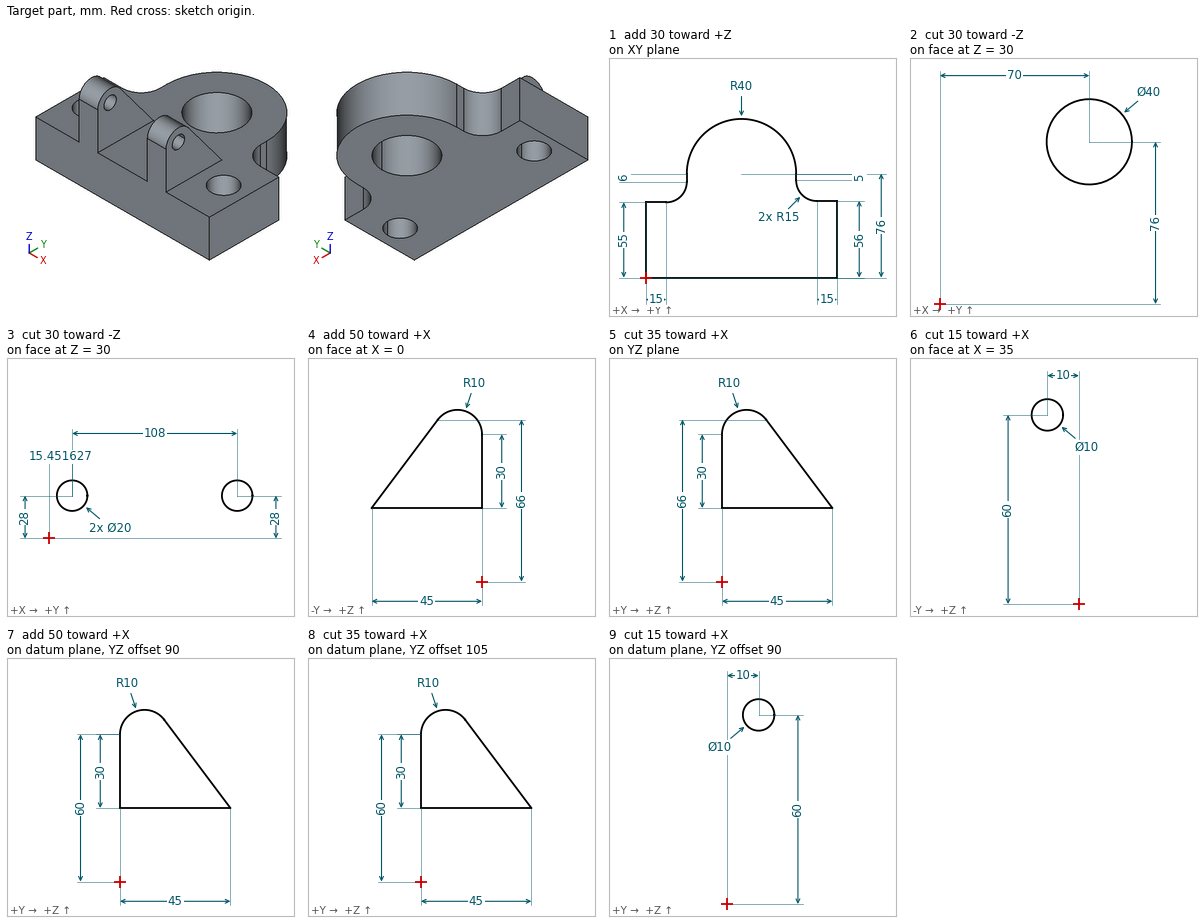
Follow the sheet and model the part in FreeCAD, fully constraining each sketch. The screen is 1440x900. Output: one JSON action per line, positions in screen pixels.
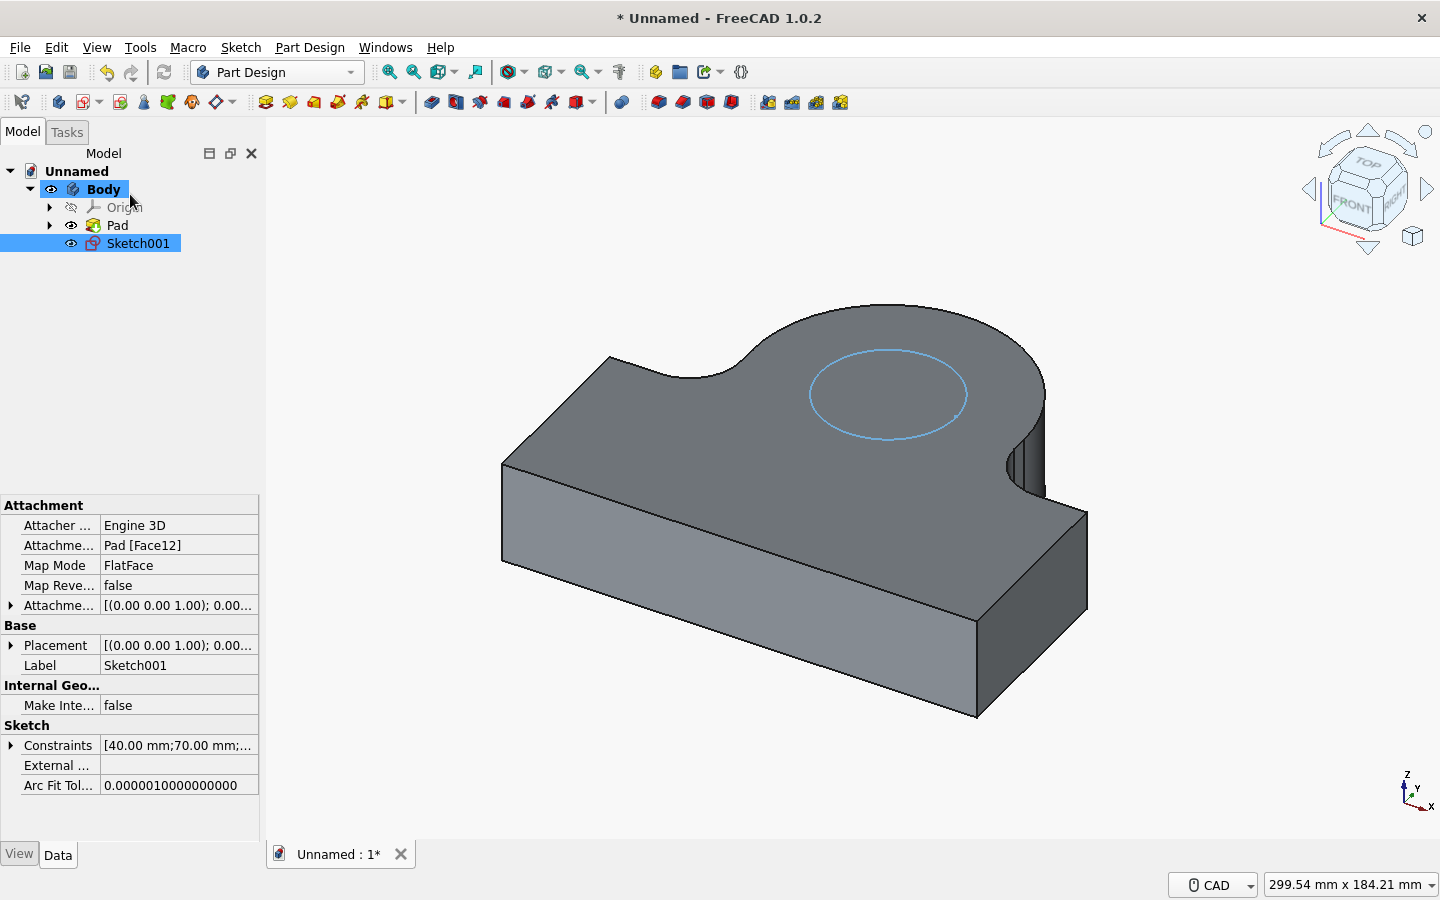
{"action": "left_click", "coordinate": [432, 102]}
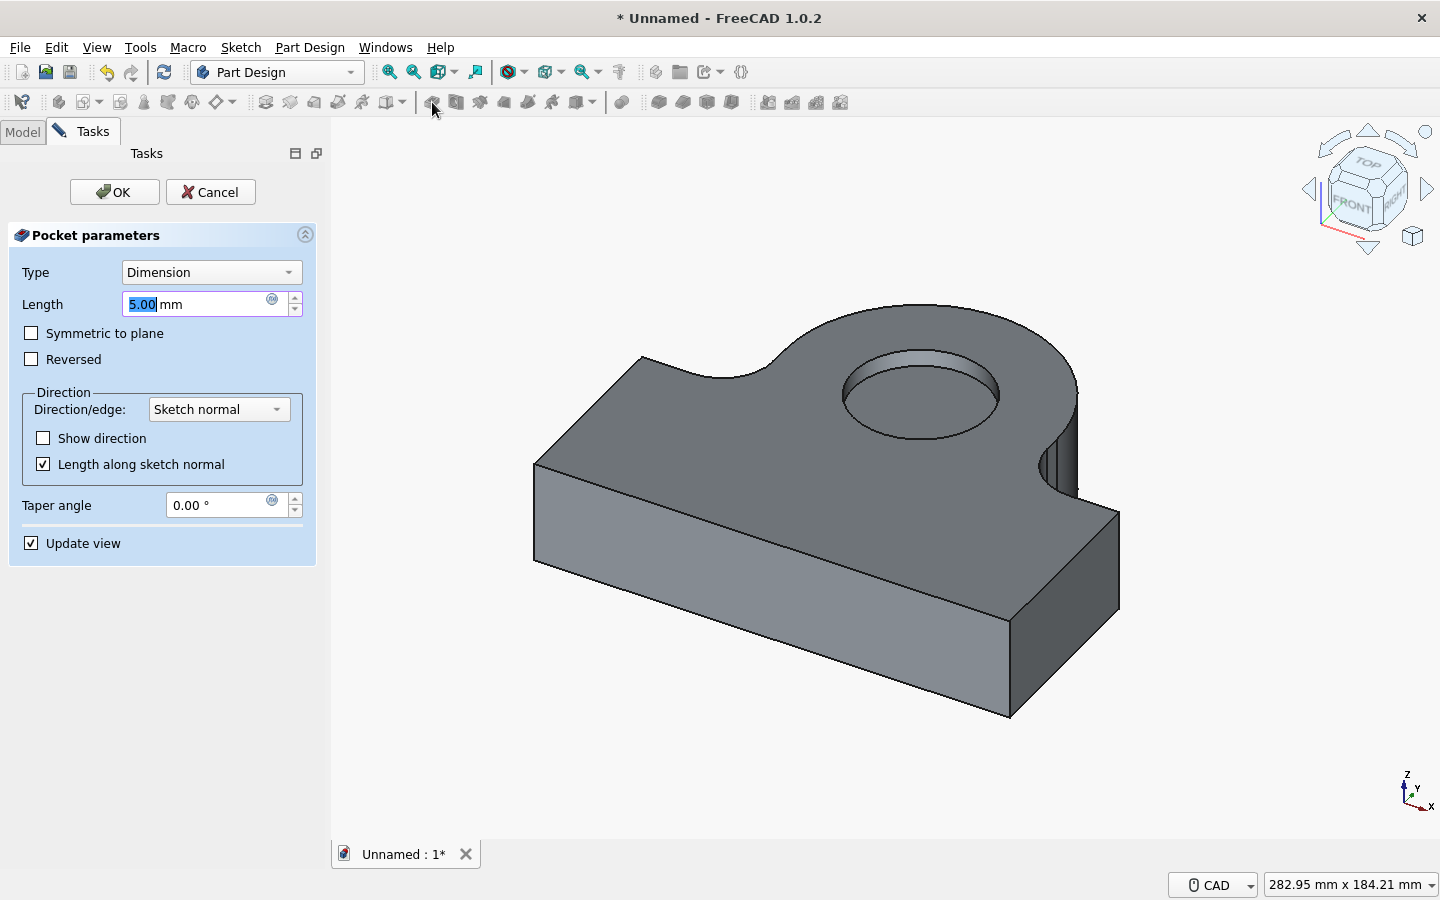
{"action": "type", "text": "30"}
{"action": "key", "text": "Tab"}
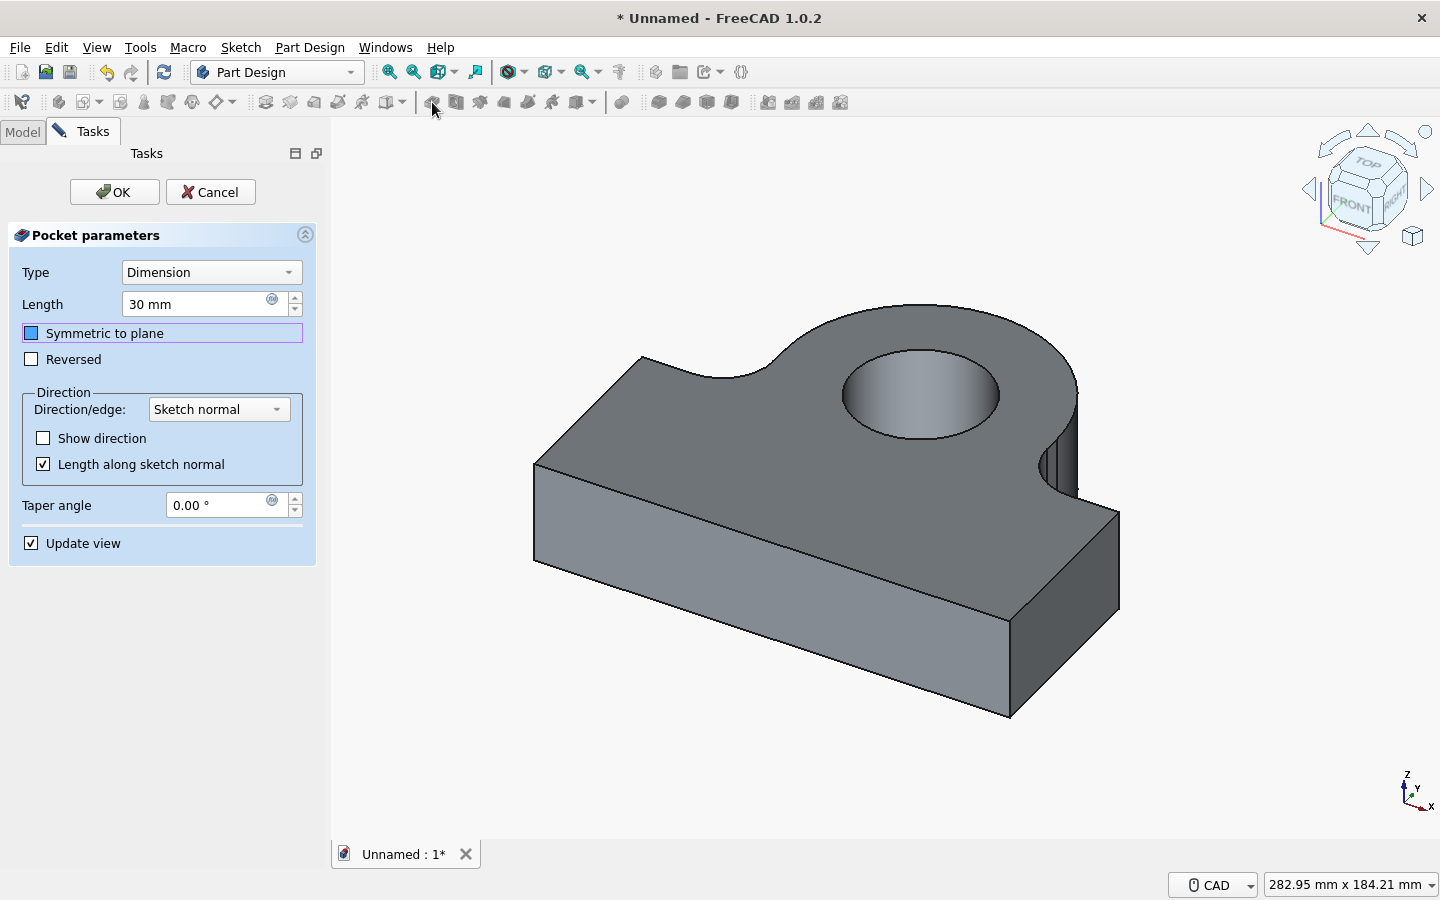
{"action": "left_click", "coordinate": [115, 192]}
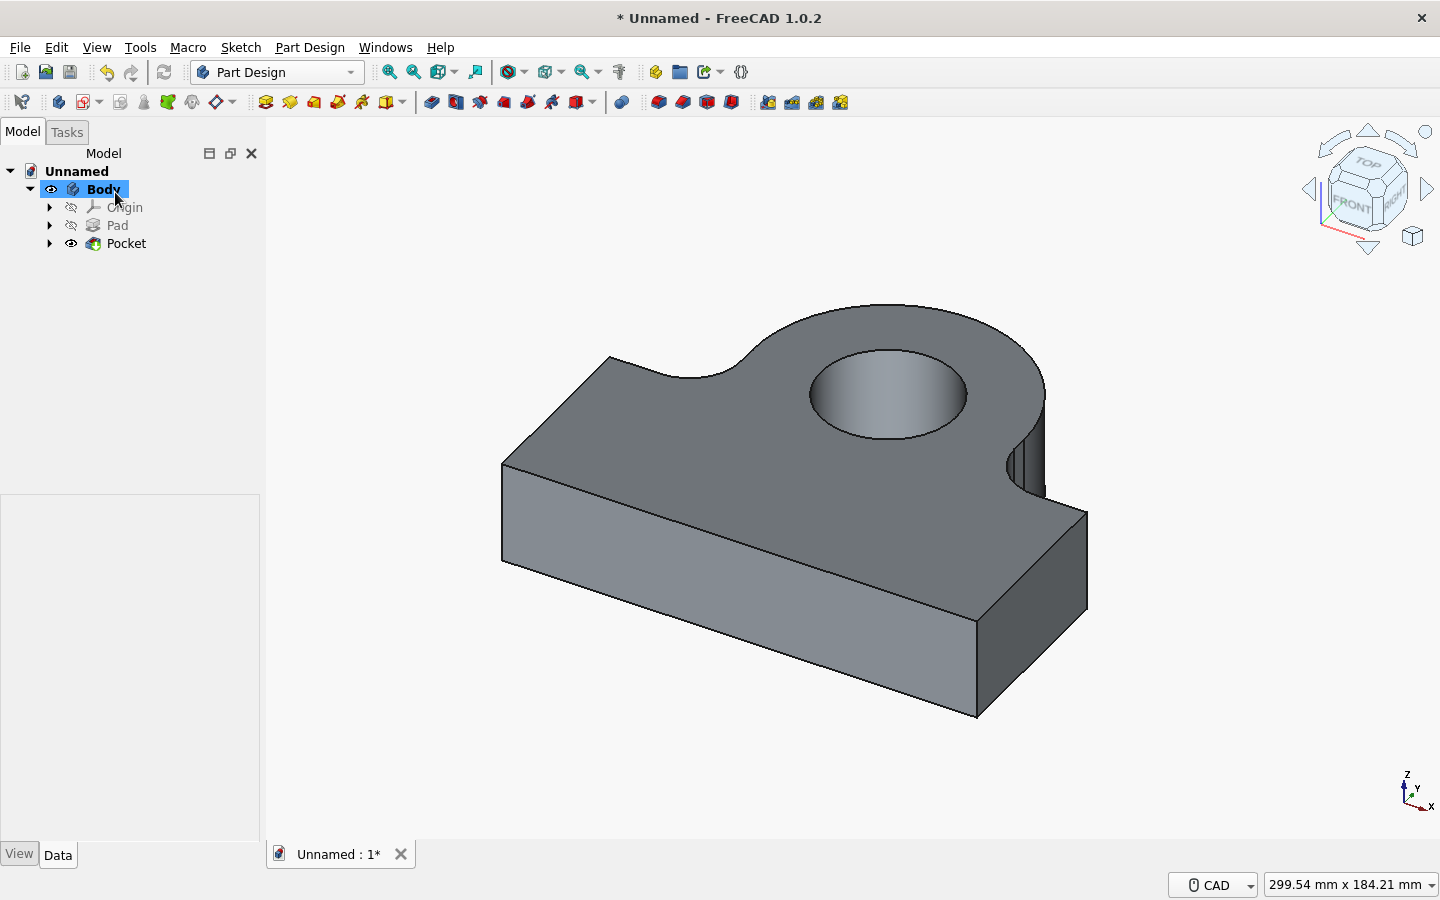
{"action": "left_click", "coordinate": [924, 538]}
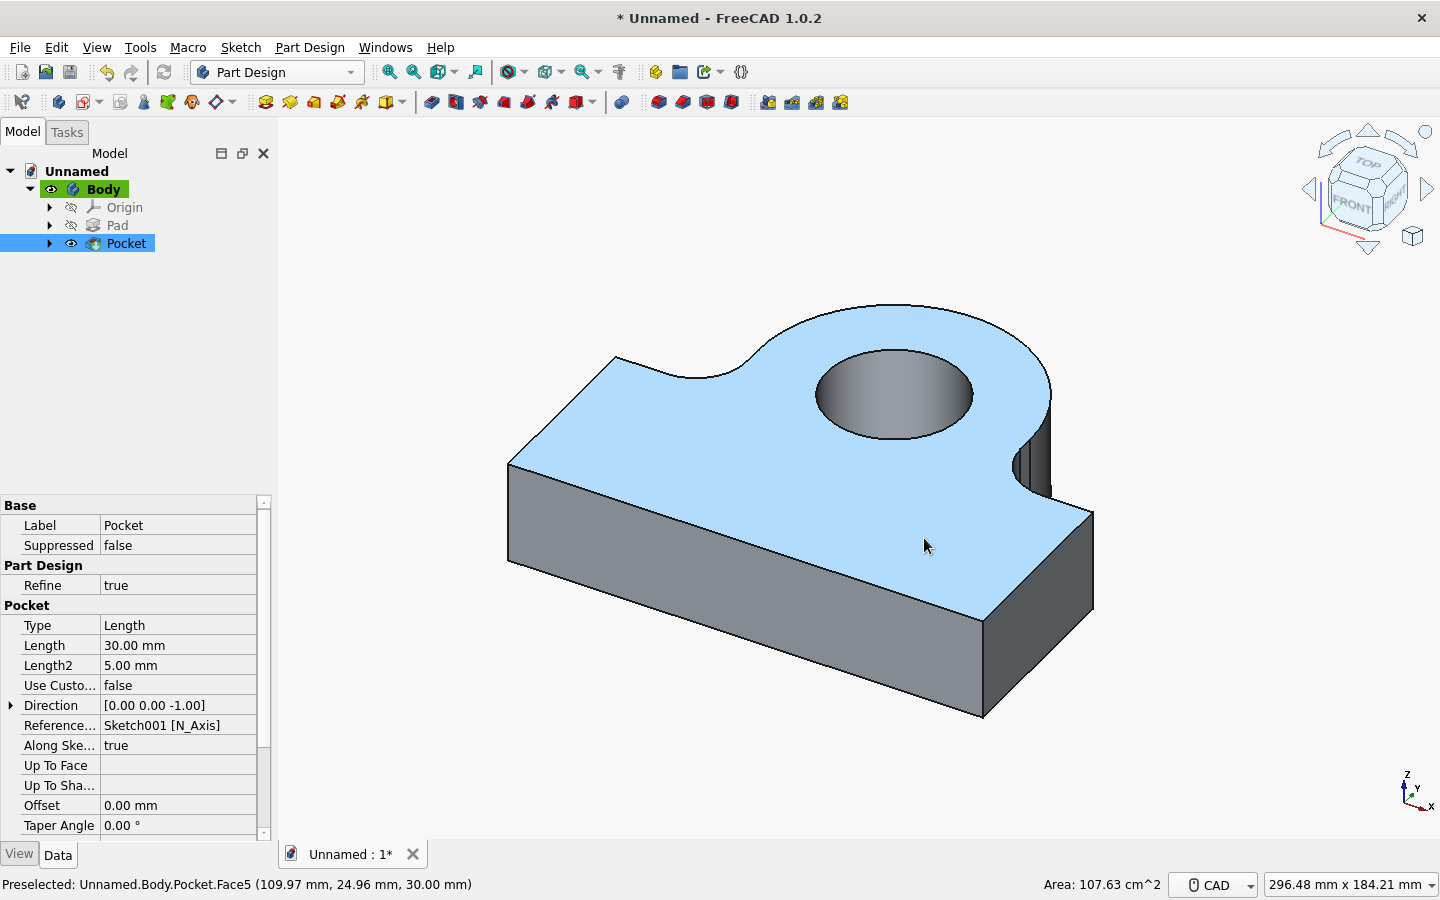
{"action": "left_click", "coordinate": [84, 102]}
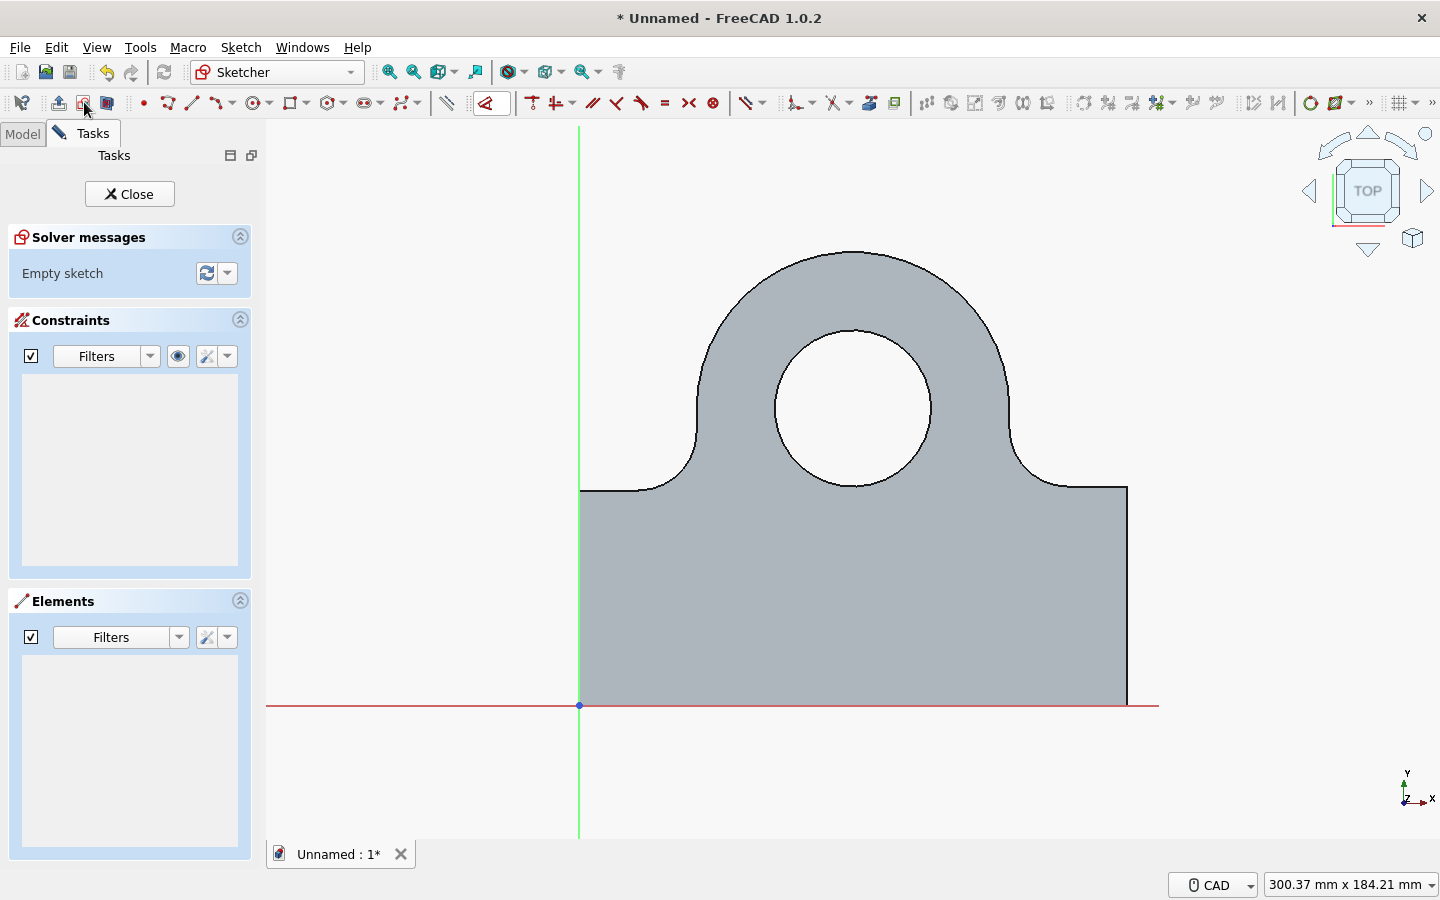
{"action": "key", "text": "g c"}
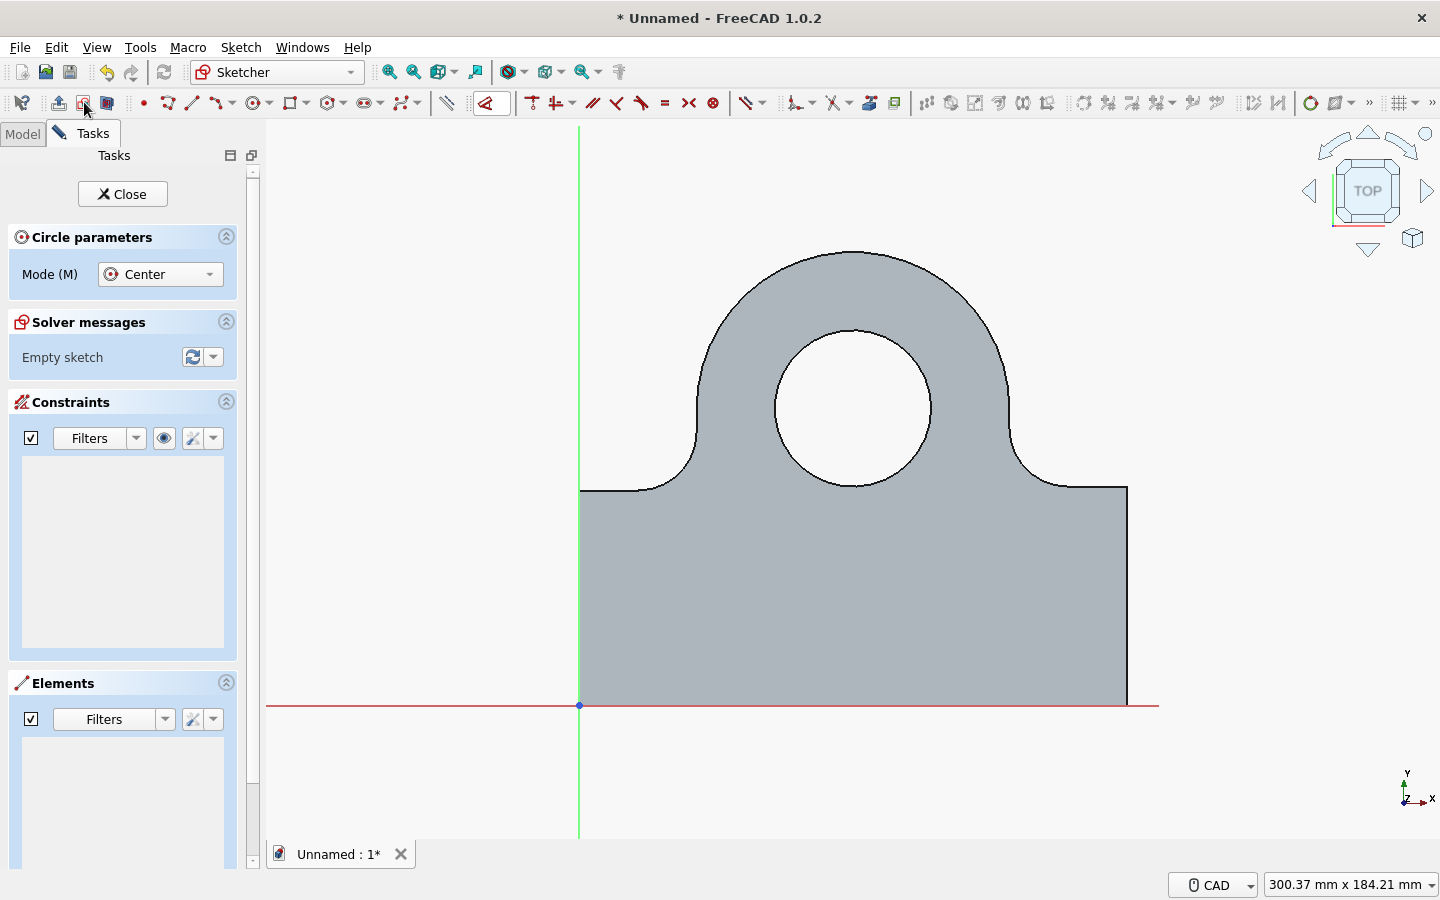
{"action": "left_click", "coordinate": [640, 596]}
{"action": "mouse_move", "coordinate": [667, 568]}